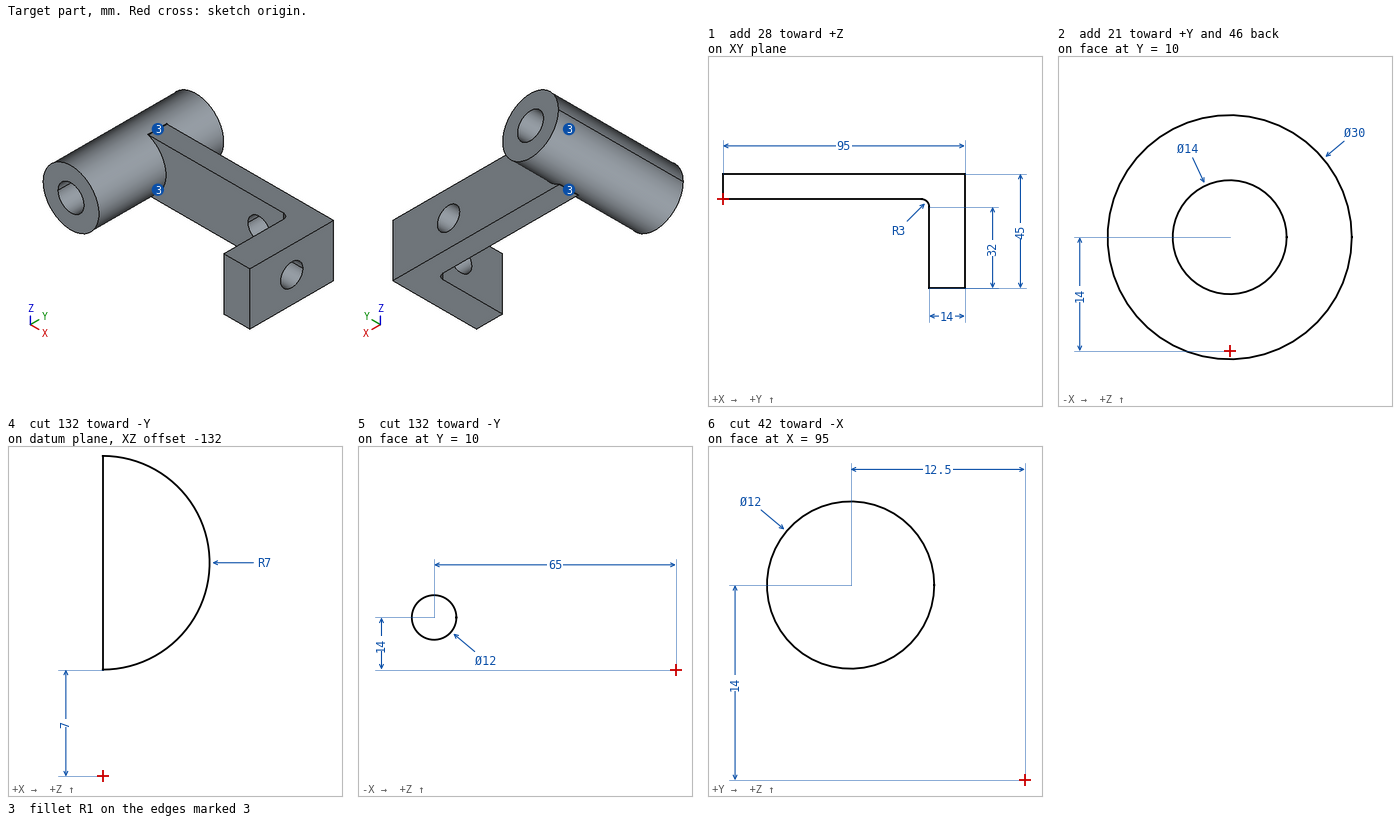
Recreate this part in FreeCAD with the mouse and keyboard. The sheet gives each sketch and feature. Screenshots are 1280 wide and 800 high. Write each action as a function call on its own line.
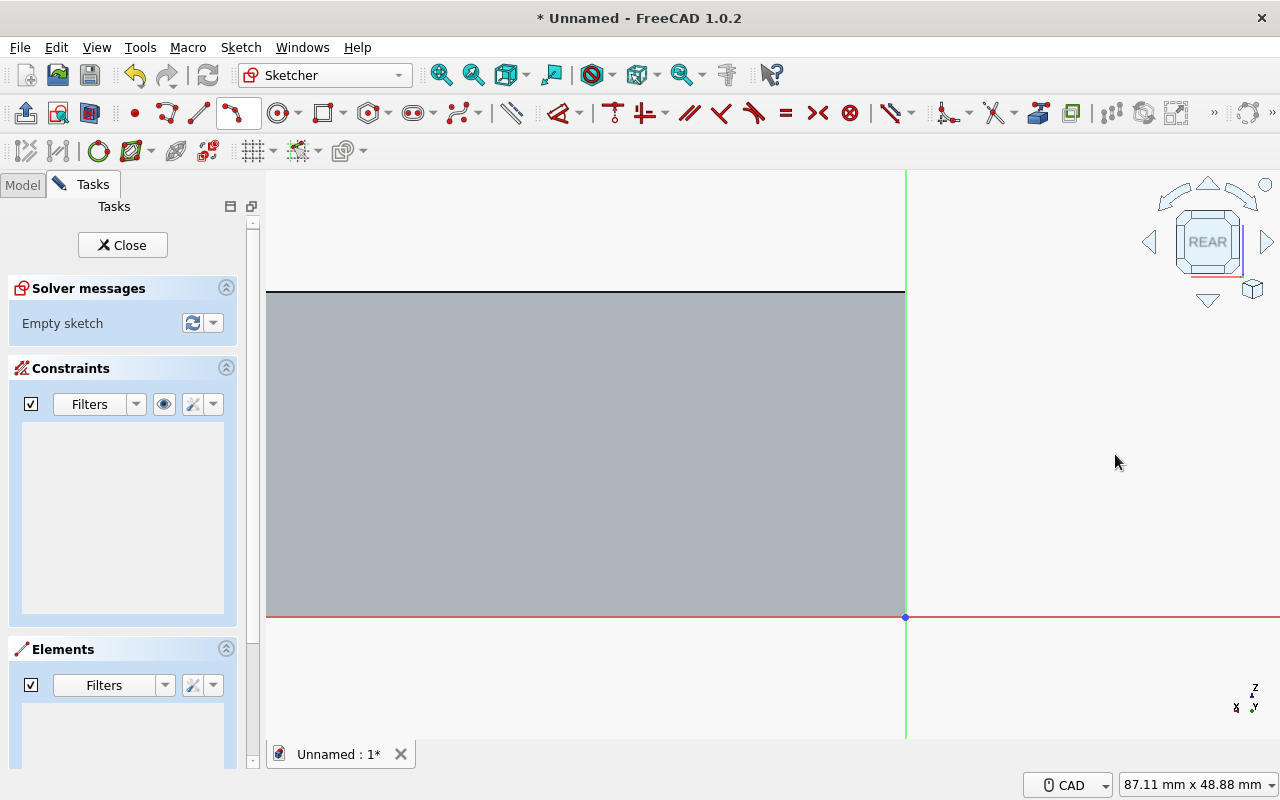
click(278, 114)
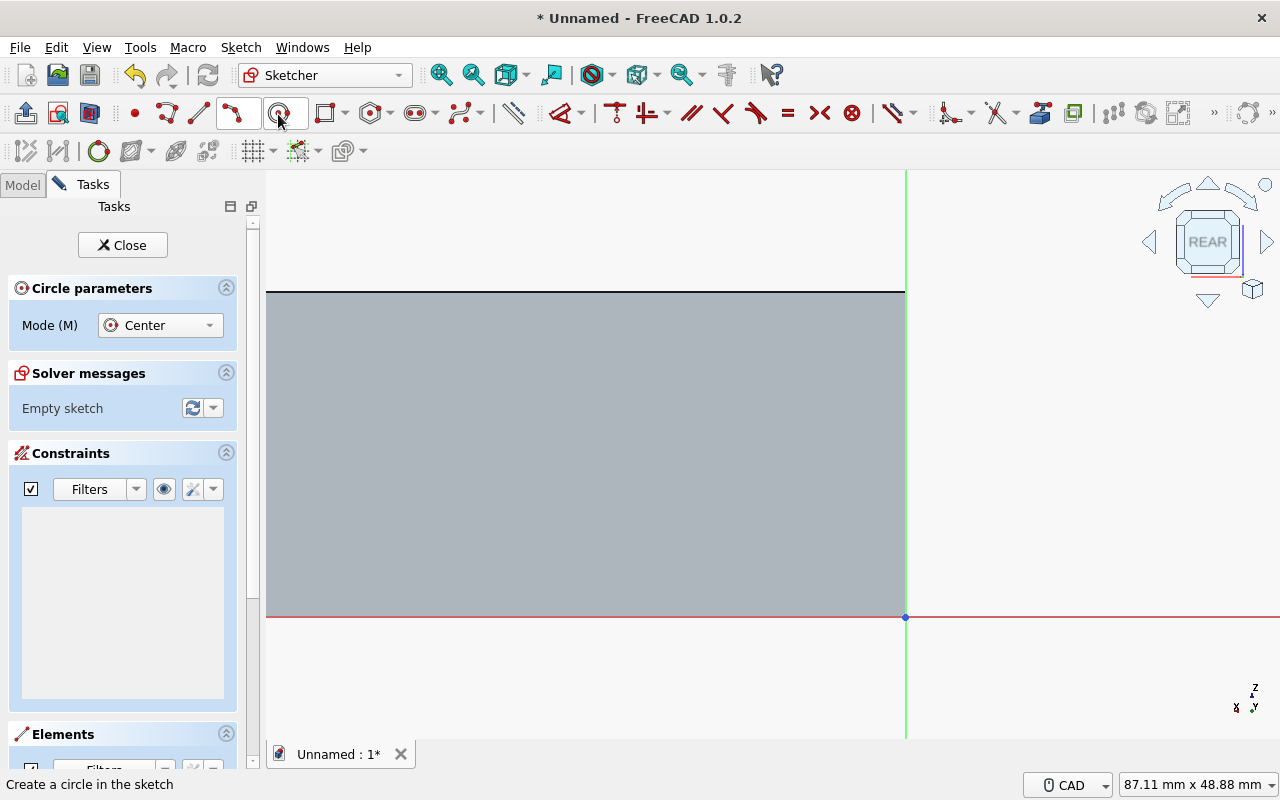
click(906, 454)
move(1029, 331)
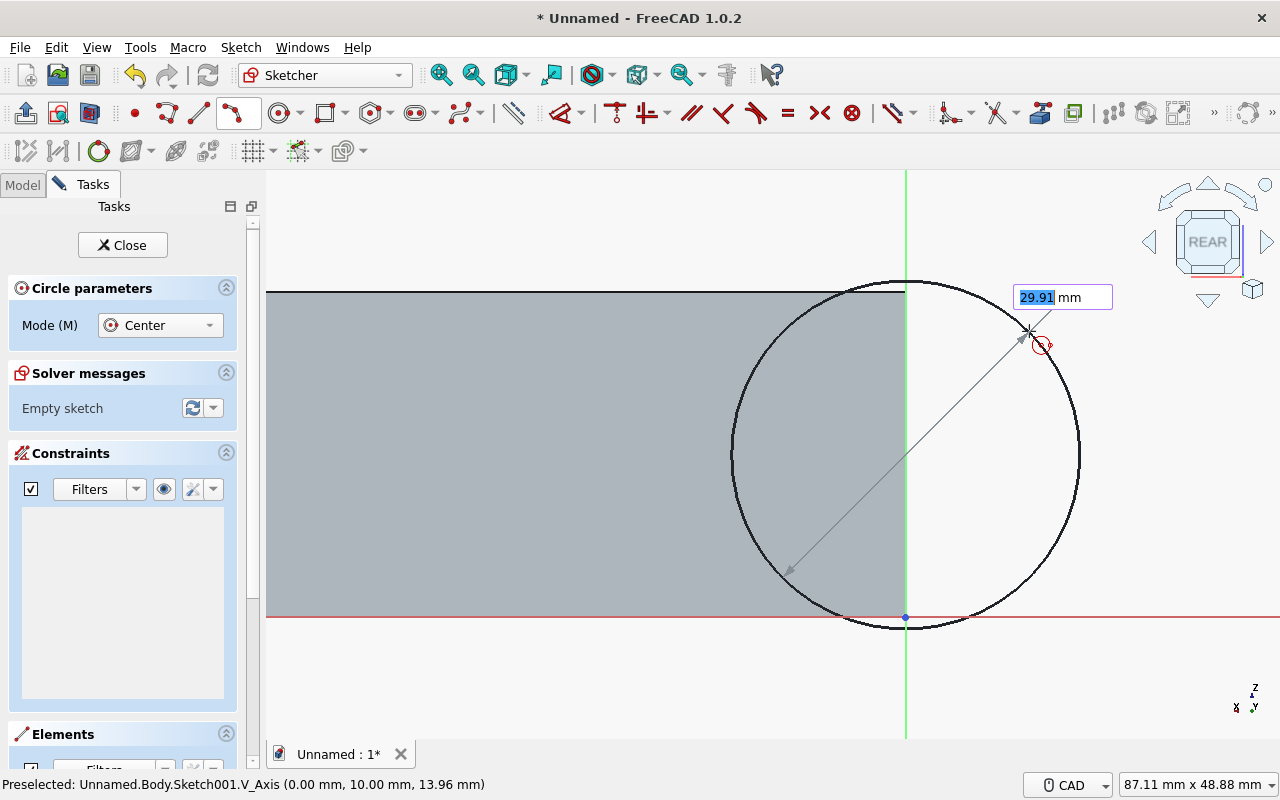
text(30)
key(Return)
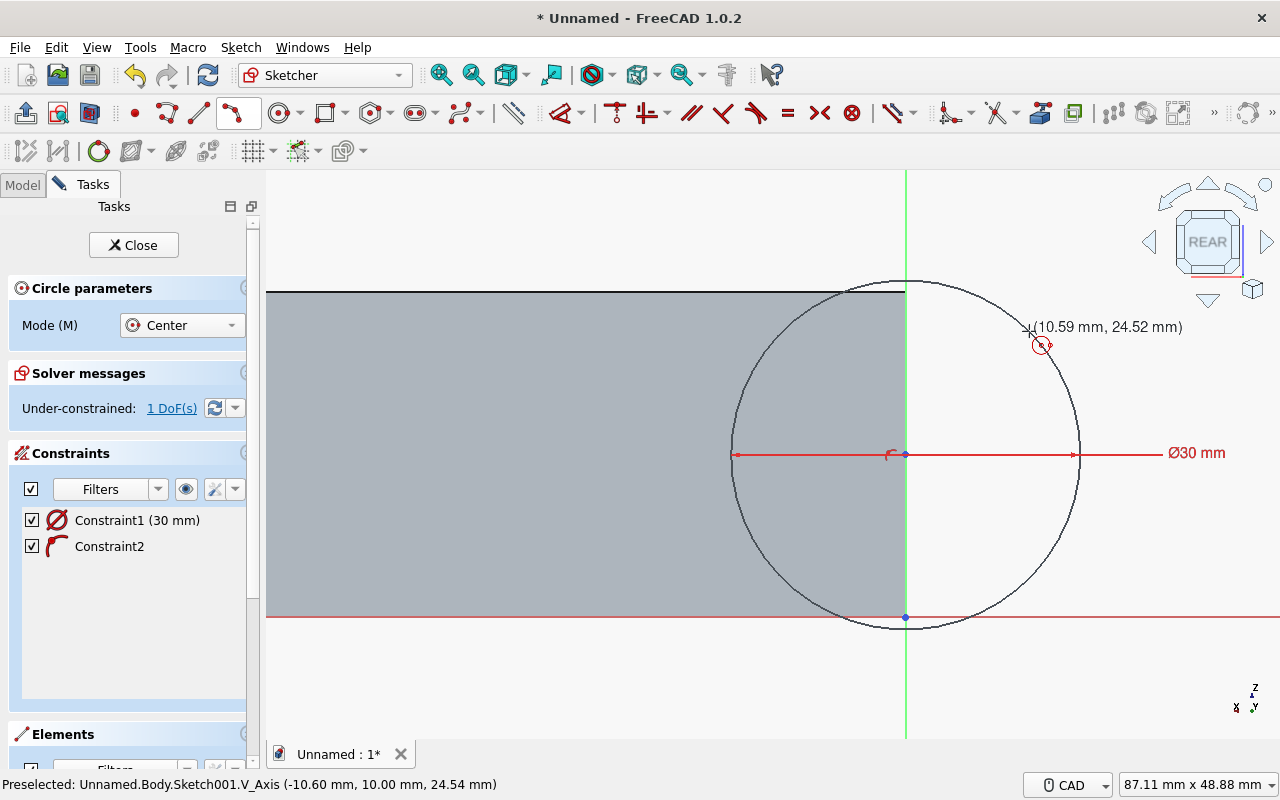
click(906, 455)
move(963, 397)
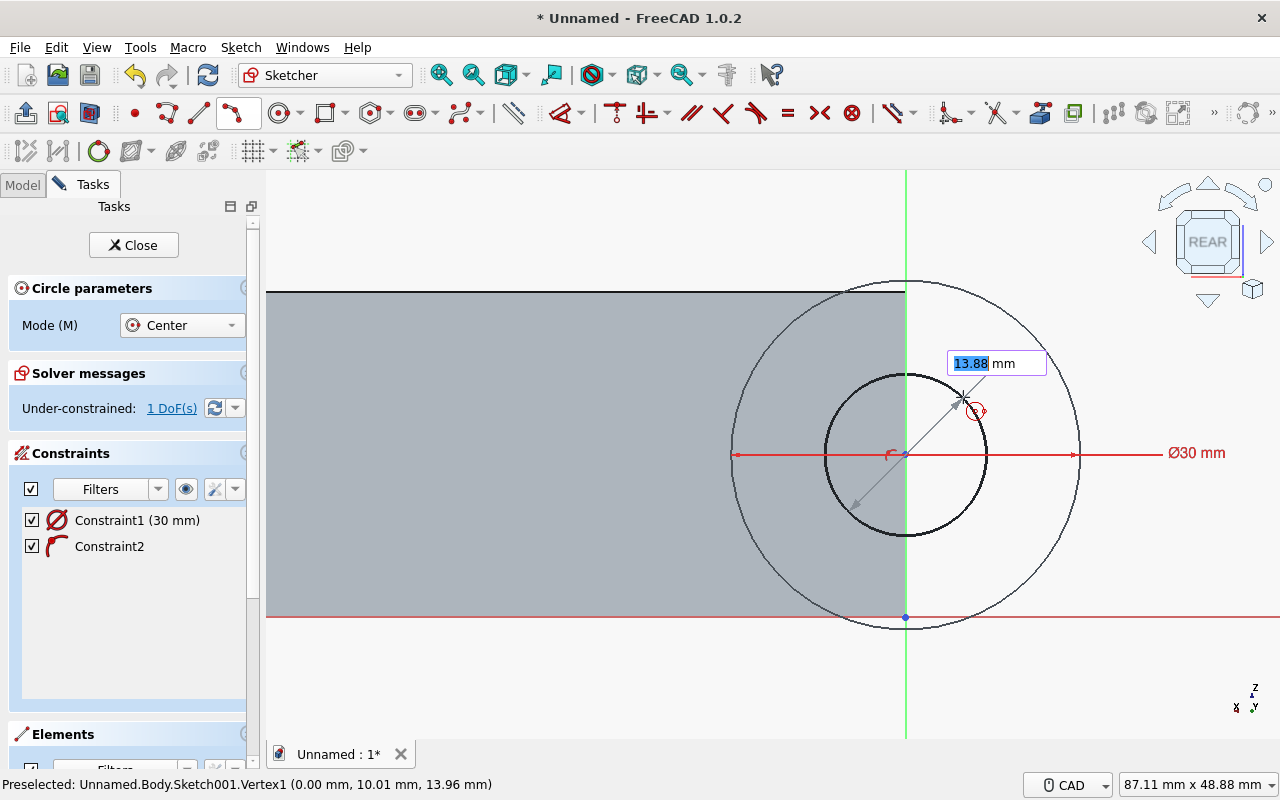
text(14)
key(Return)
key(Escape)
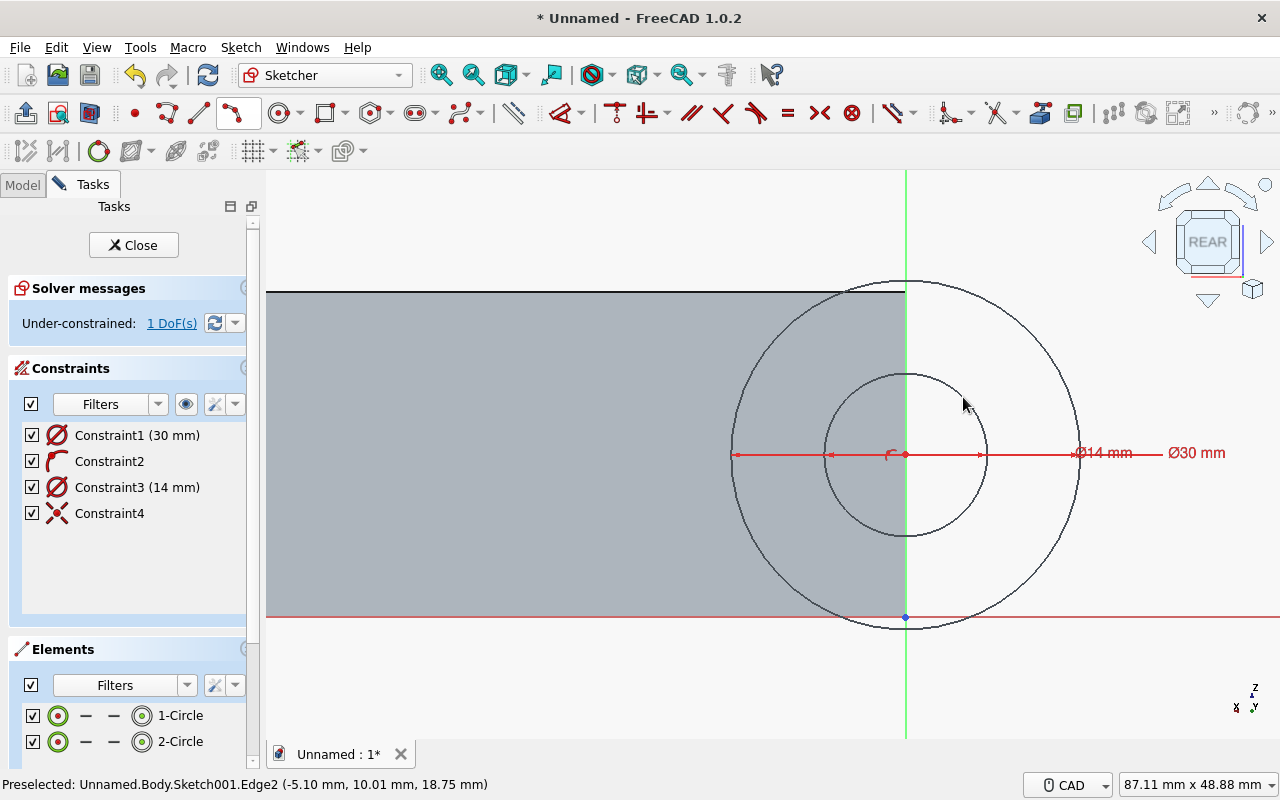
click(560, 114)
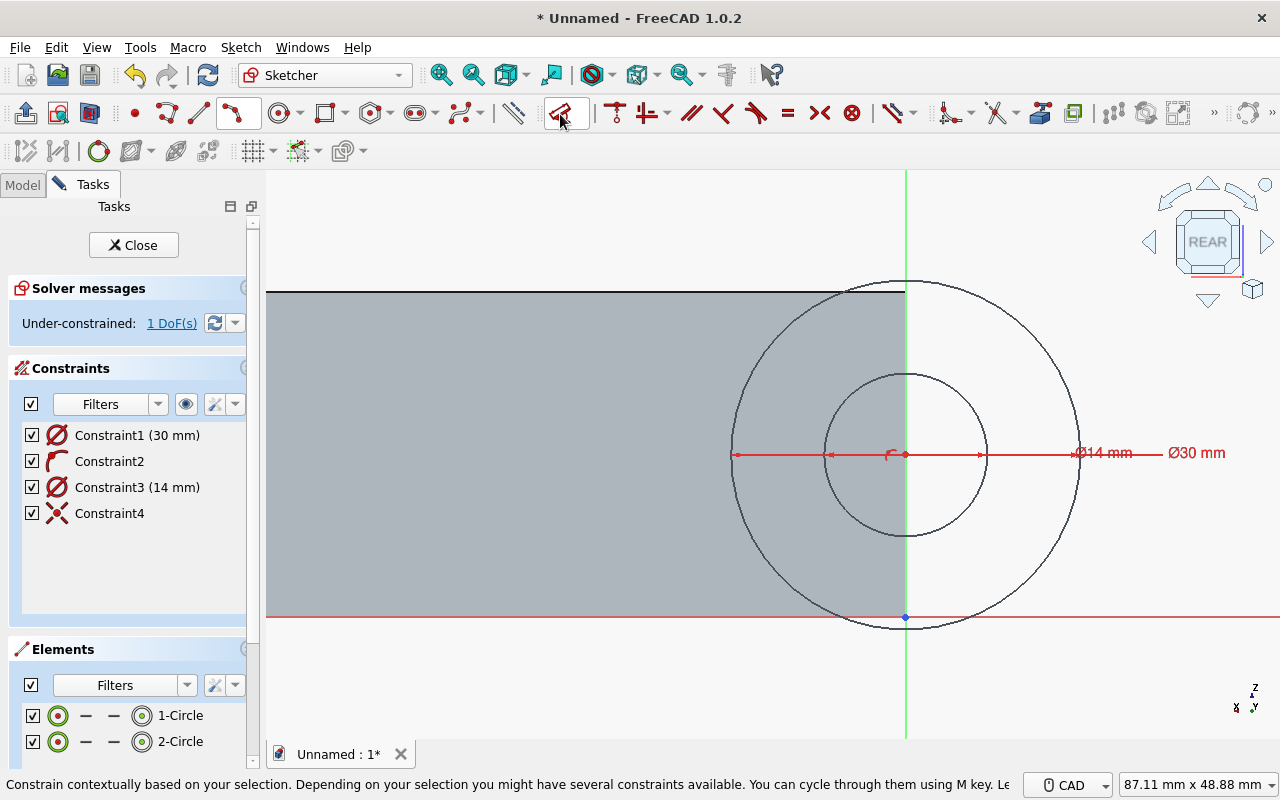
click(906, 455)
click(940, 499)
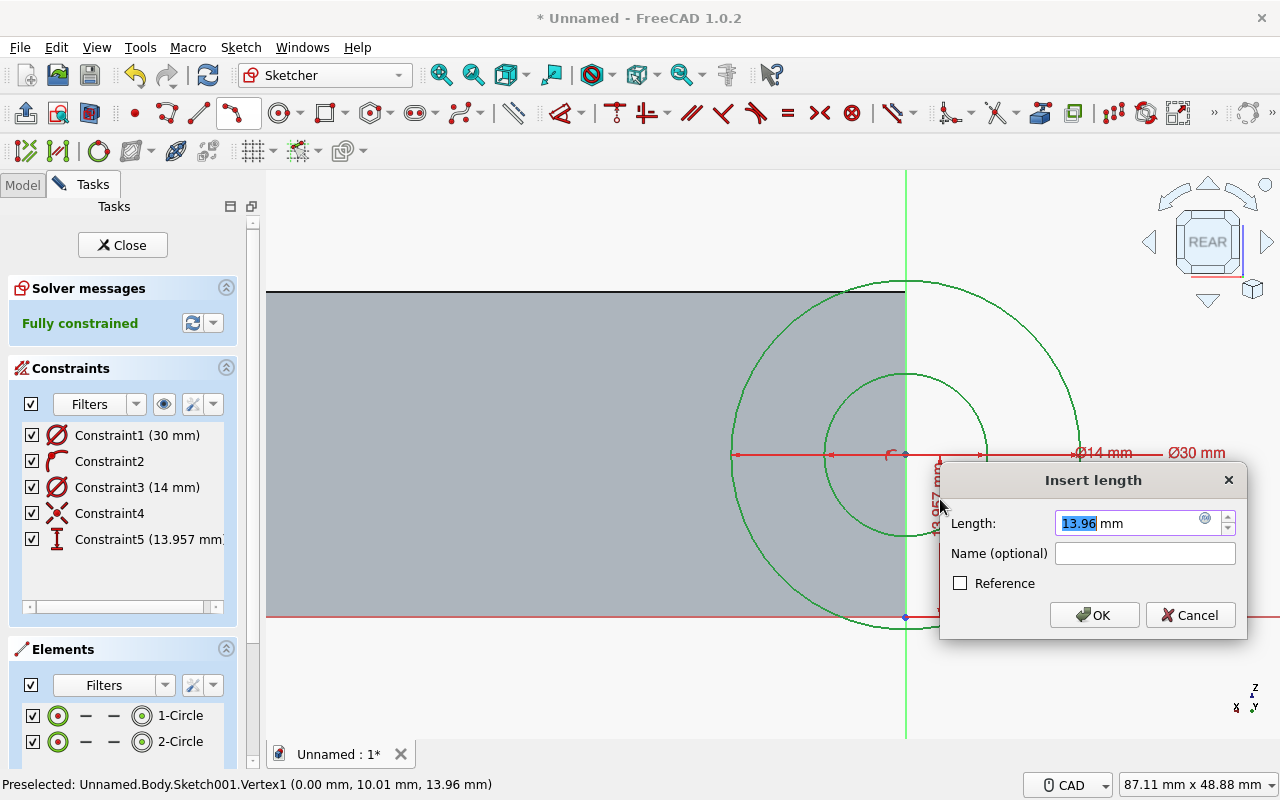
text(14)
key(Return)
key(Escape)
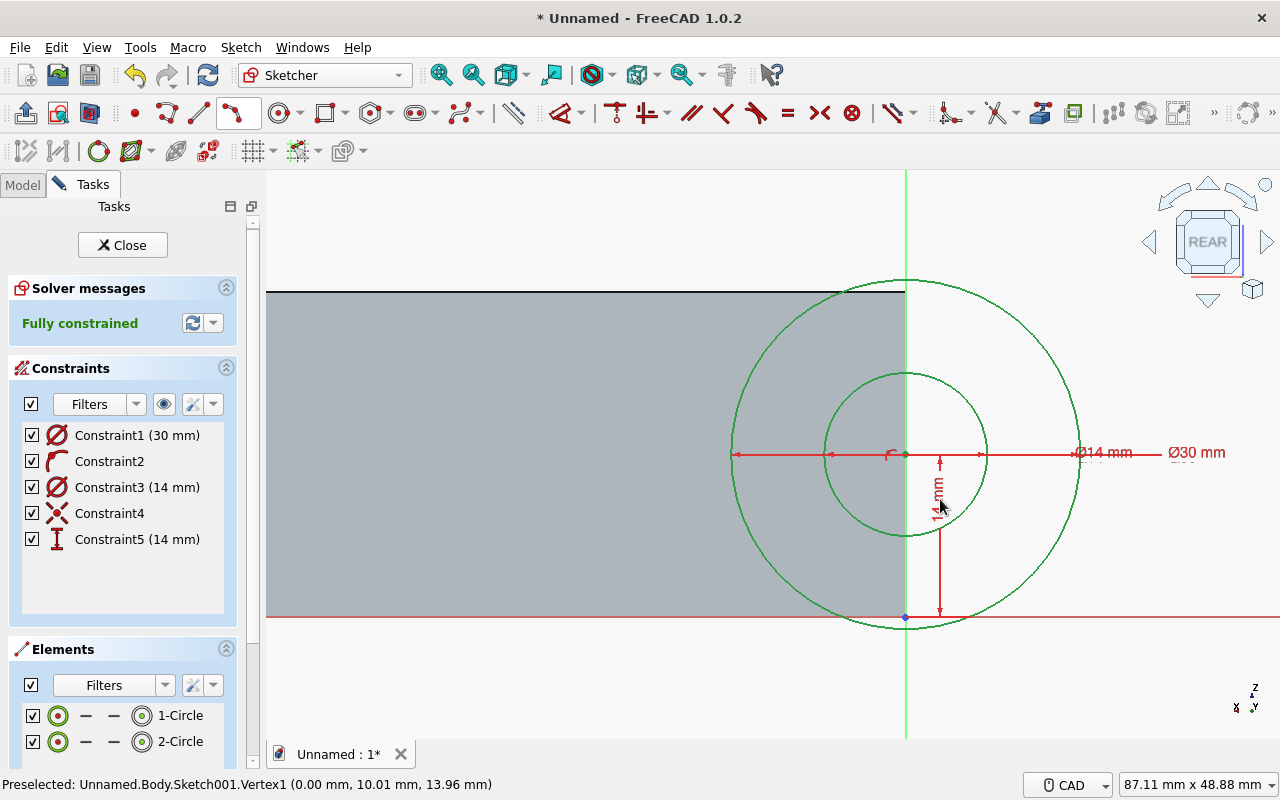
click(123, 245)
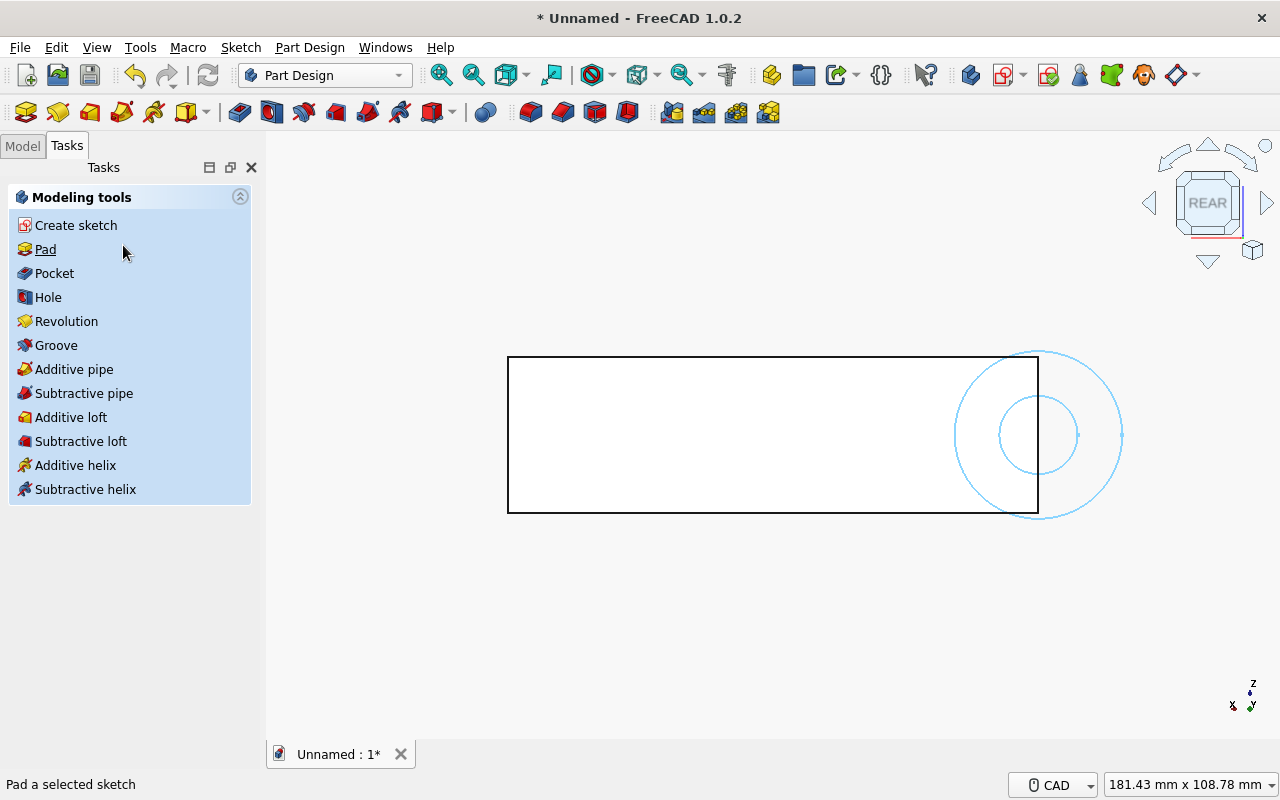
click(26, 112)